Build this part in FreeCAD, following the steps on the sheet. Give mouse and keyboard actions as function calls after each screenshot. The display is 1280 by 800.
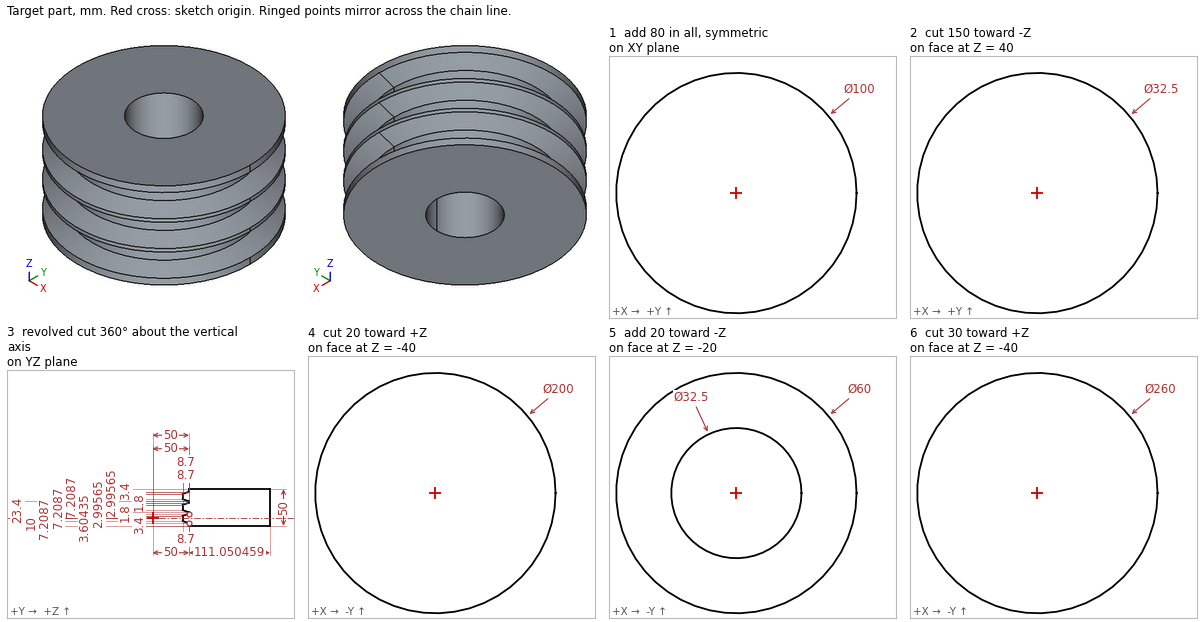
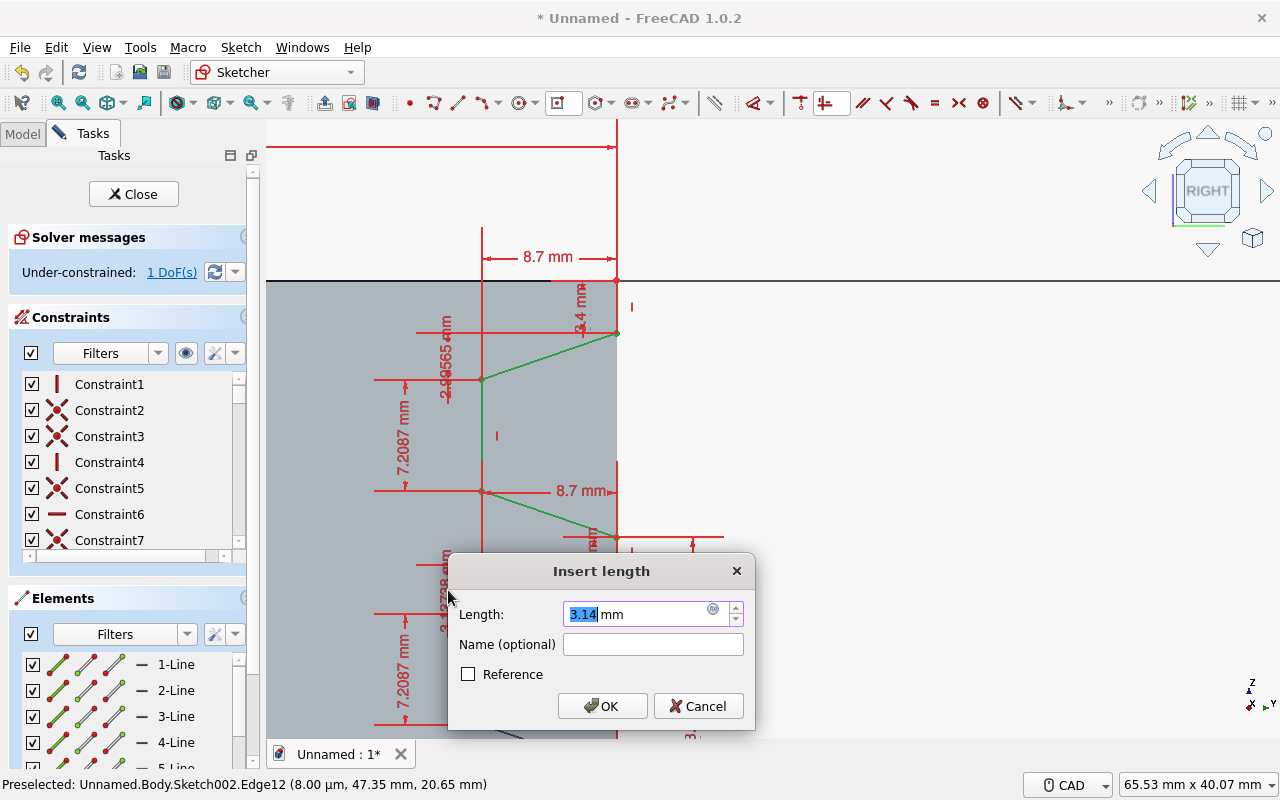
text(2.99565)
key(Return)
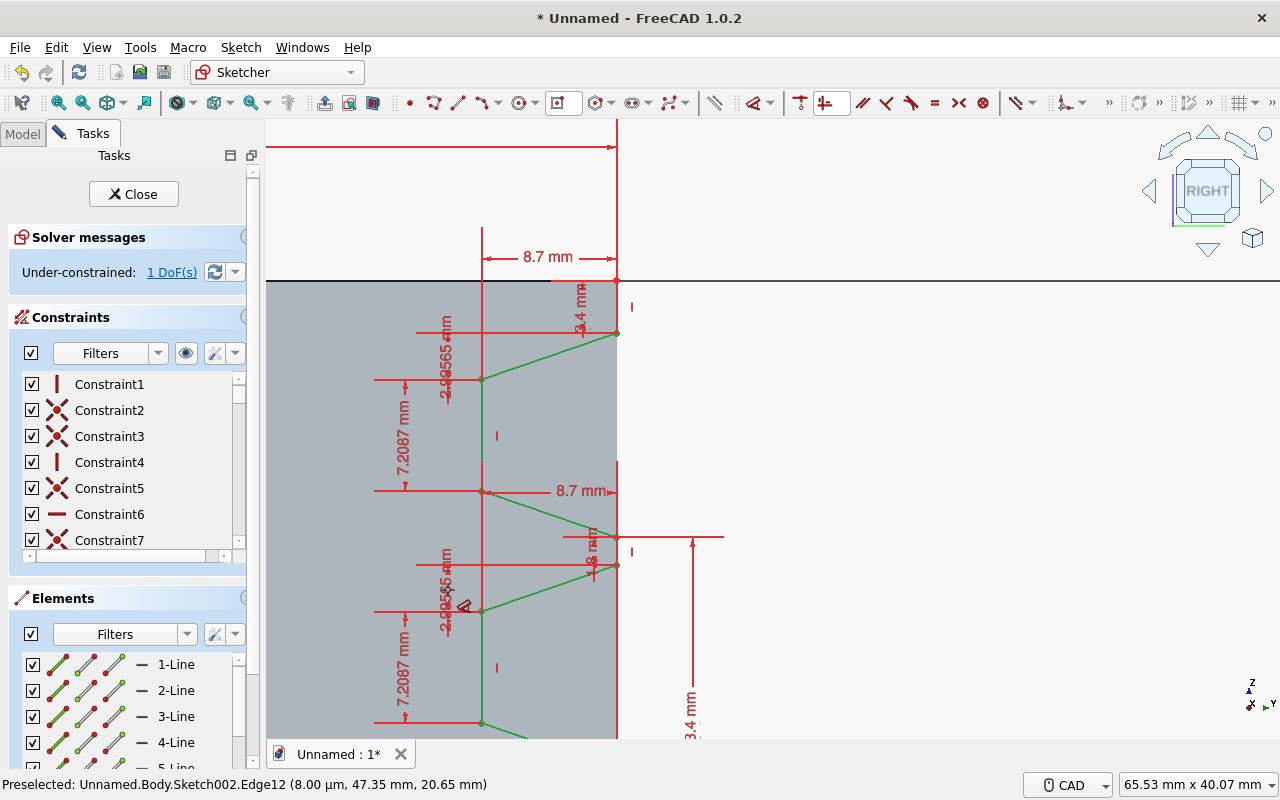
scroll(579, 351, down, 7)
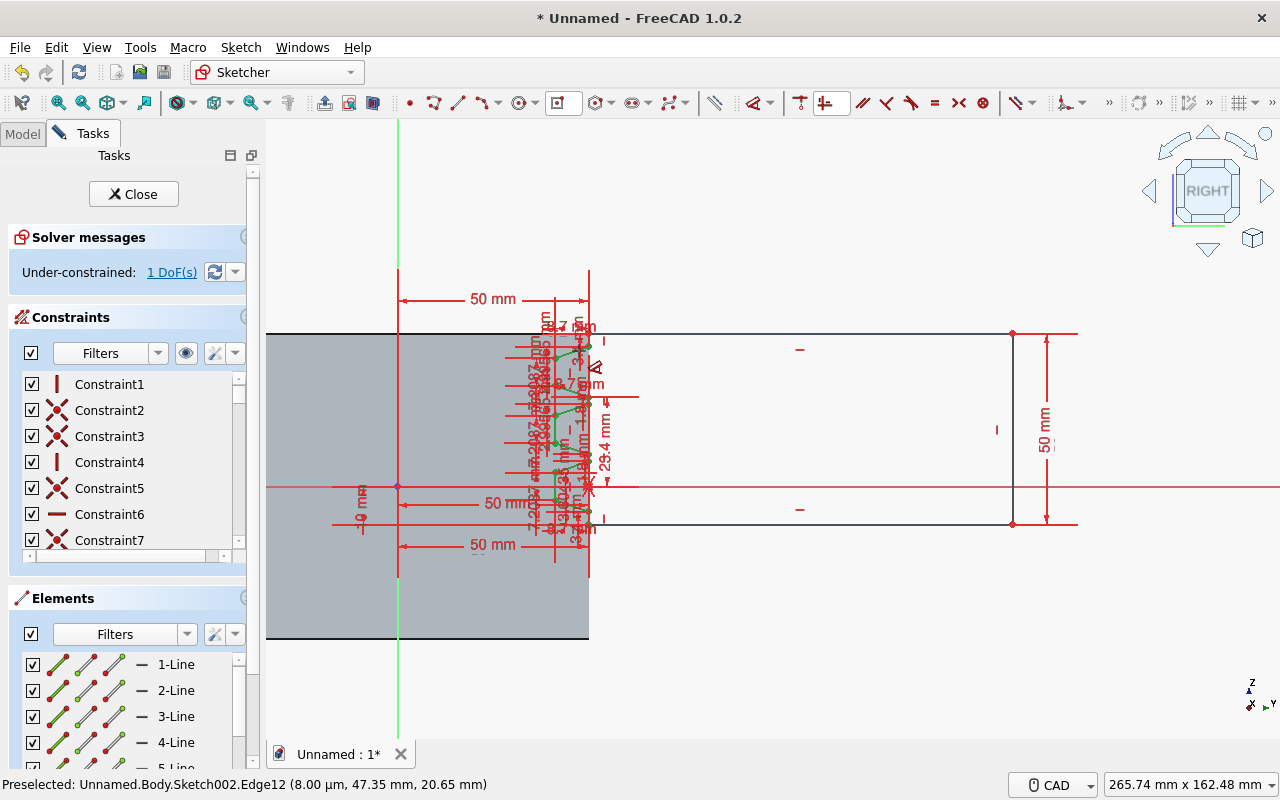
click(716, 525)
click(801, 559)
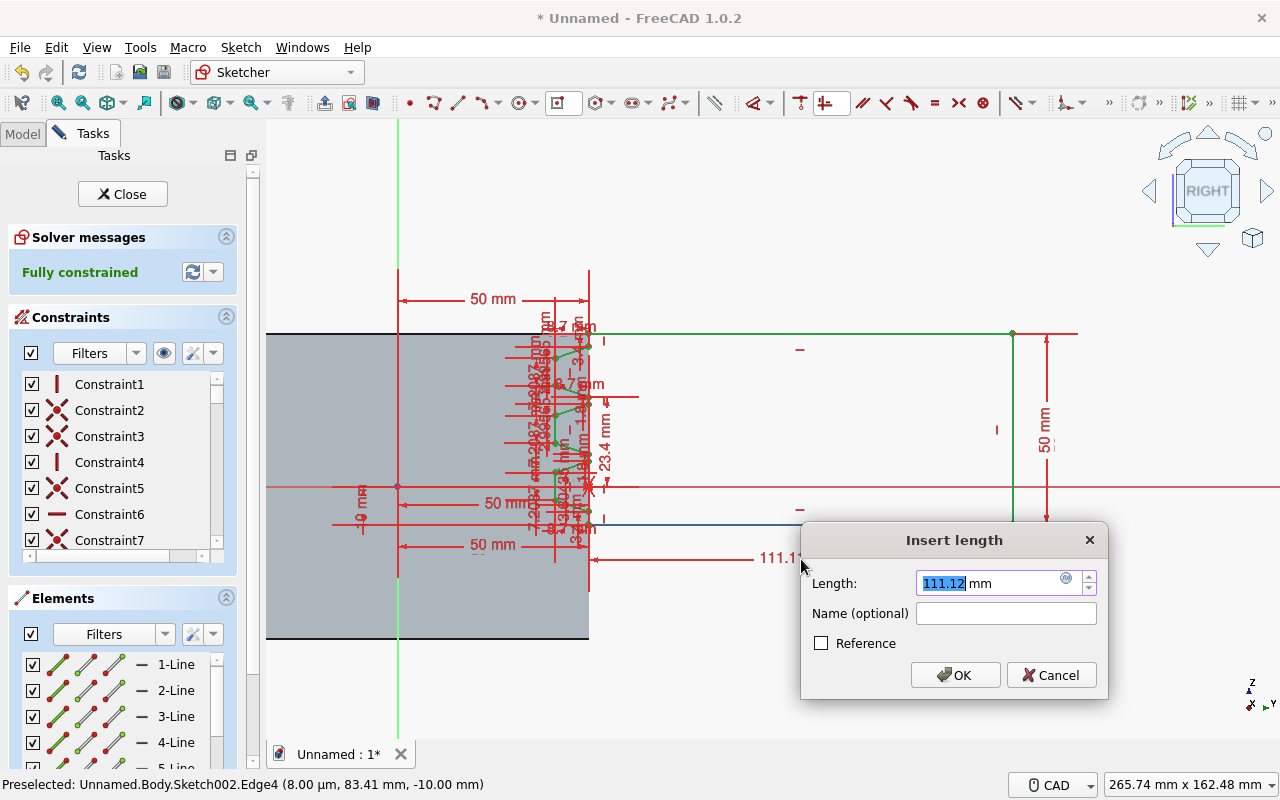
text(111.050459)
key(Return)
key(Escape)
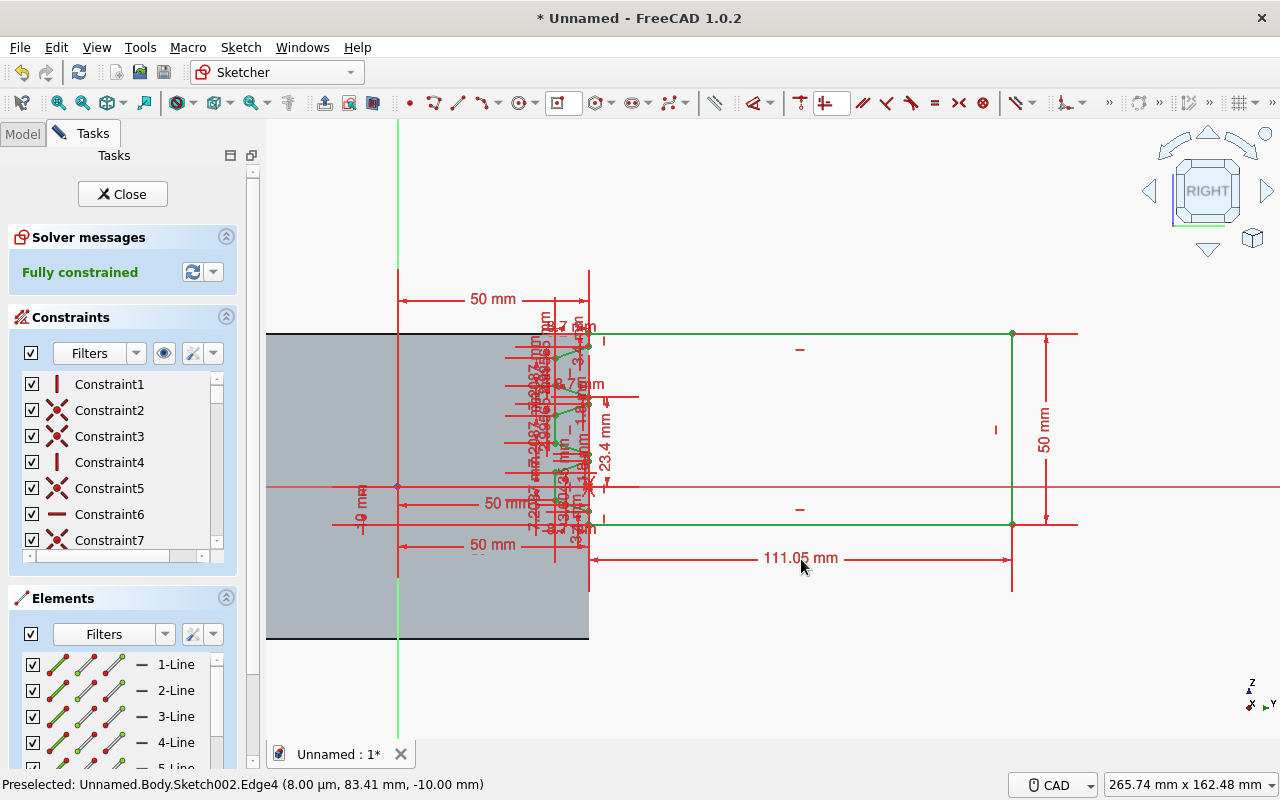
click(123, 194)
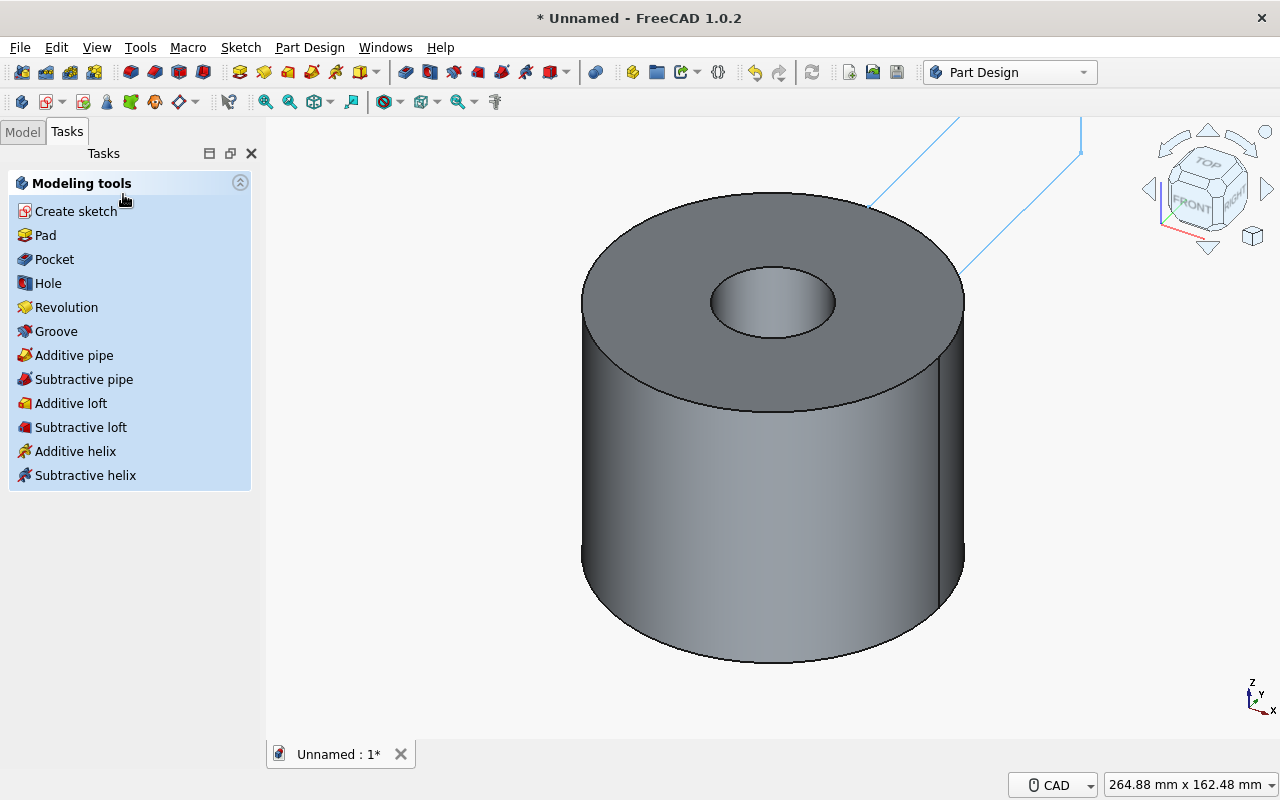
click(454, 72)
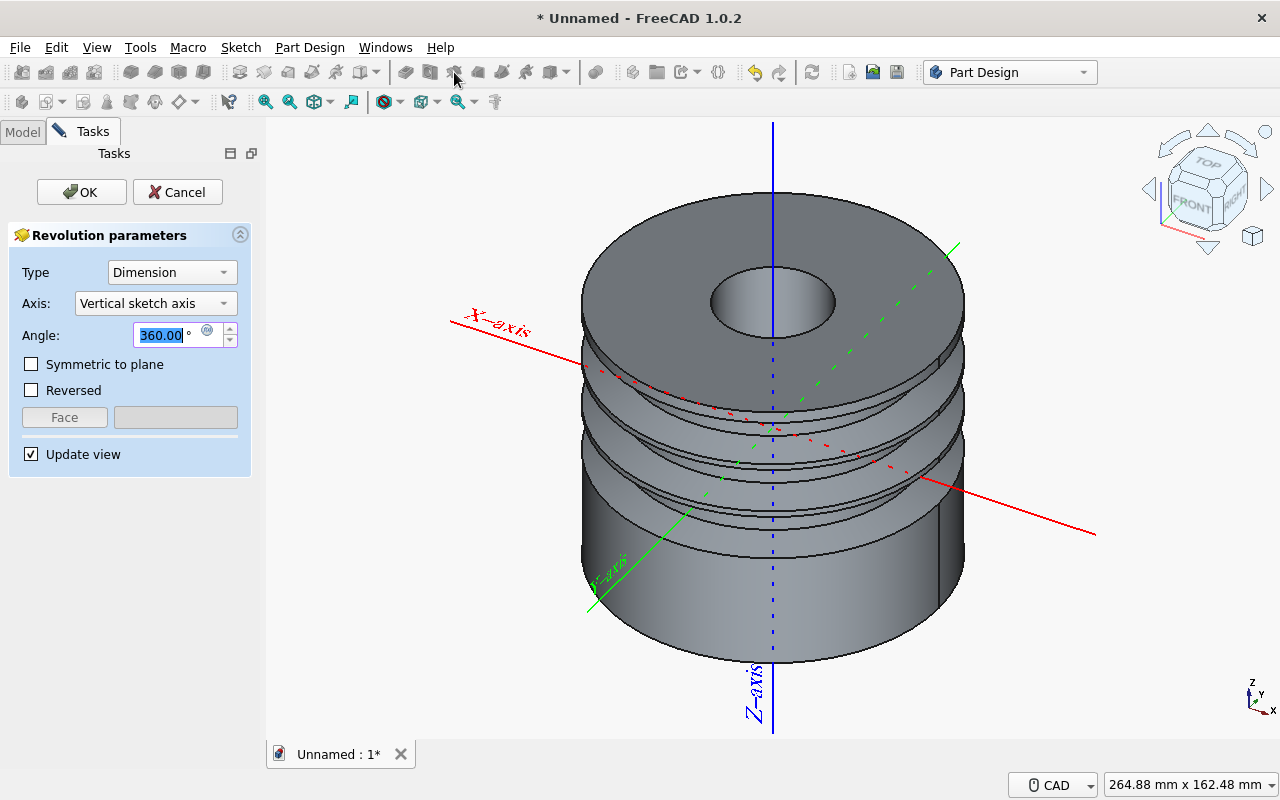
click(82, 192)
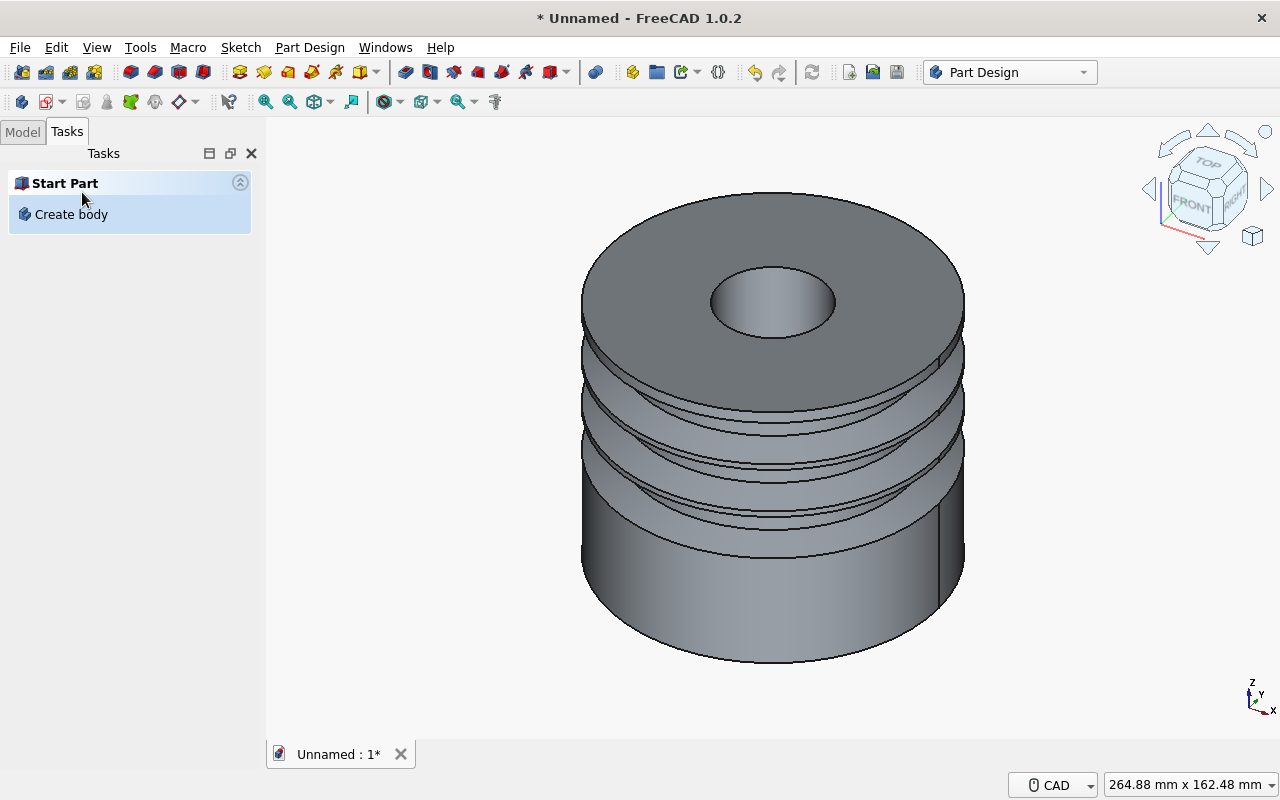
key(5)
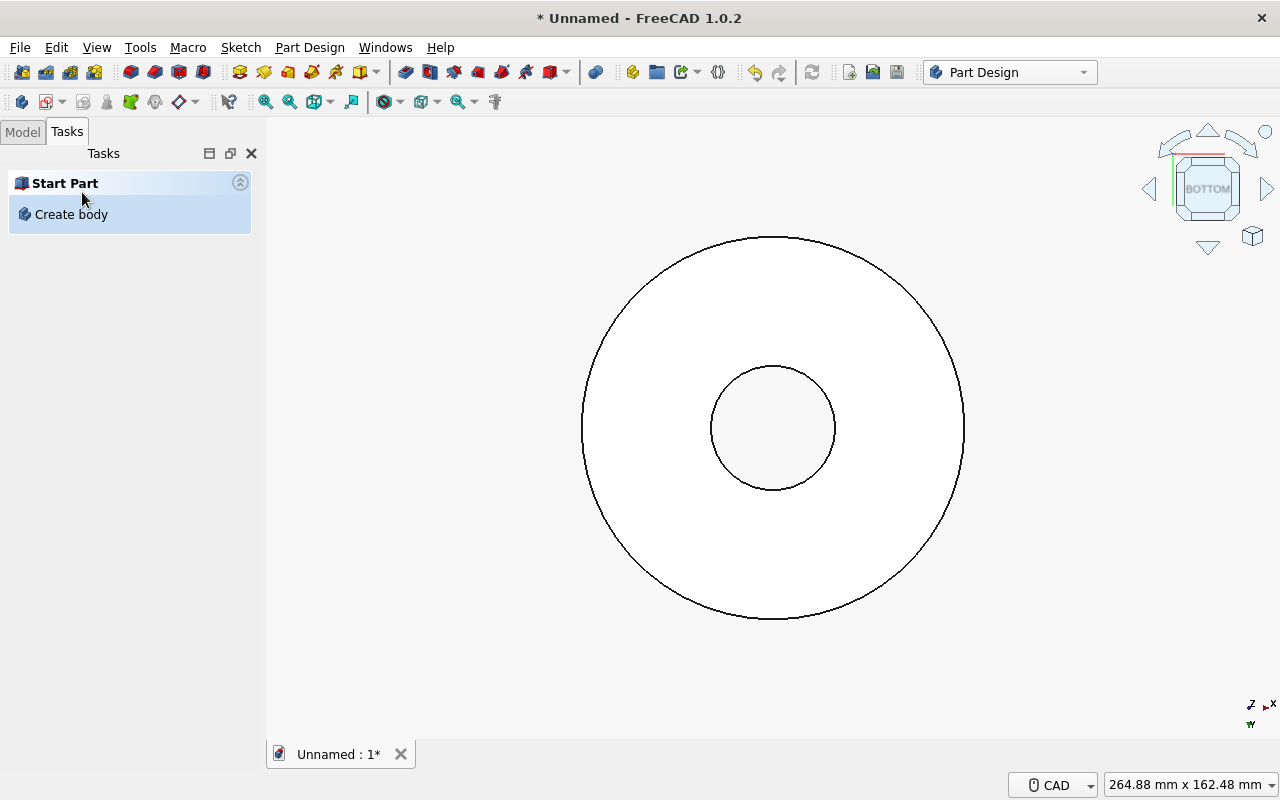
click(664, 482)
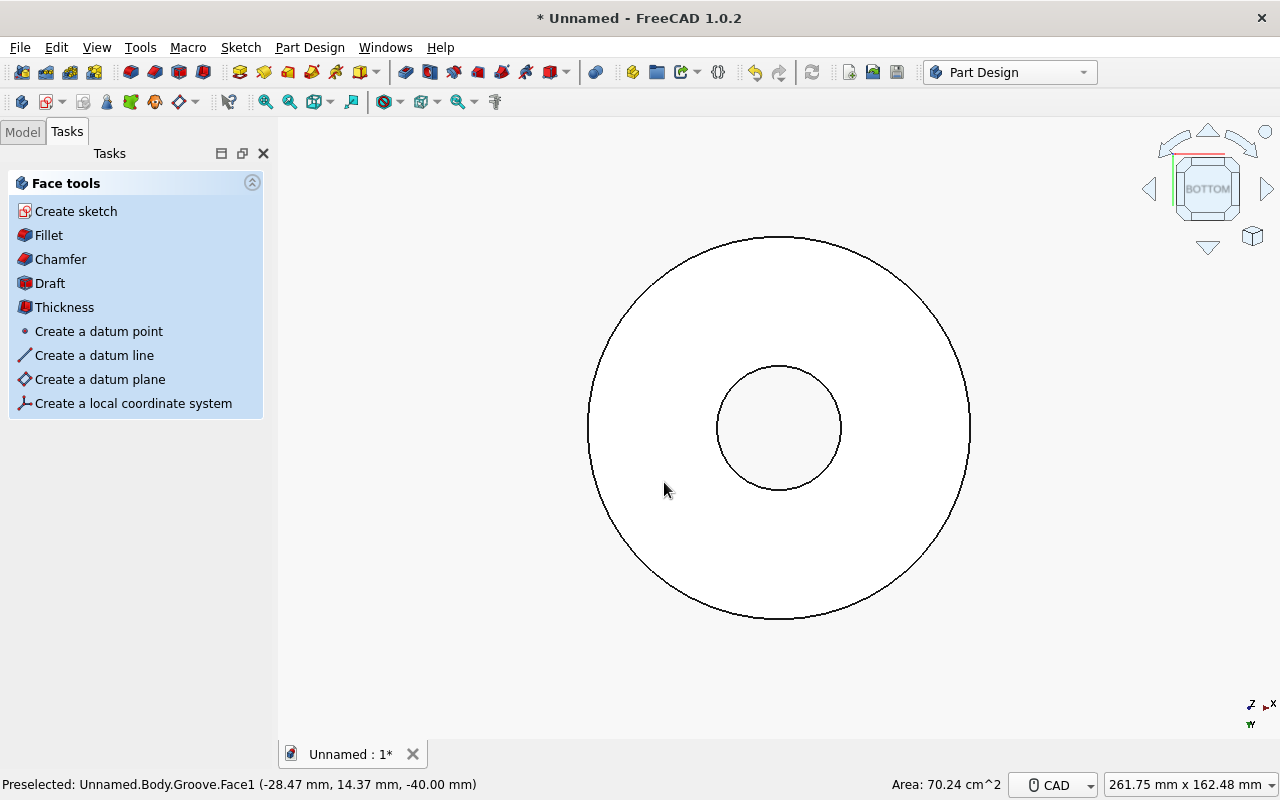
click(46, 102)